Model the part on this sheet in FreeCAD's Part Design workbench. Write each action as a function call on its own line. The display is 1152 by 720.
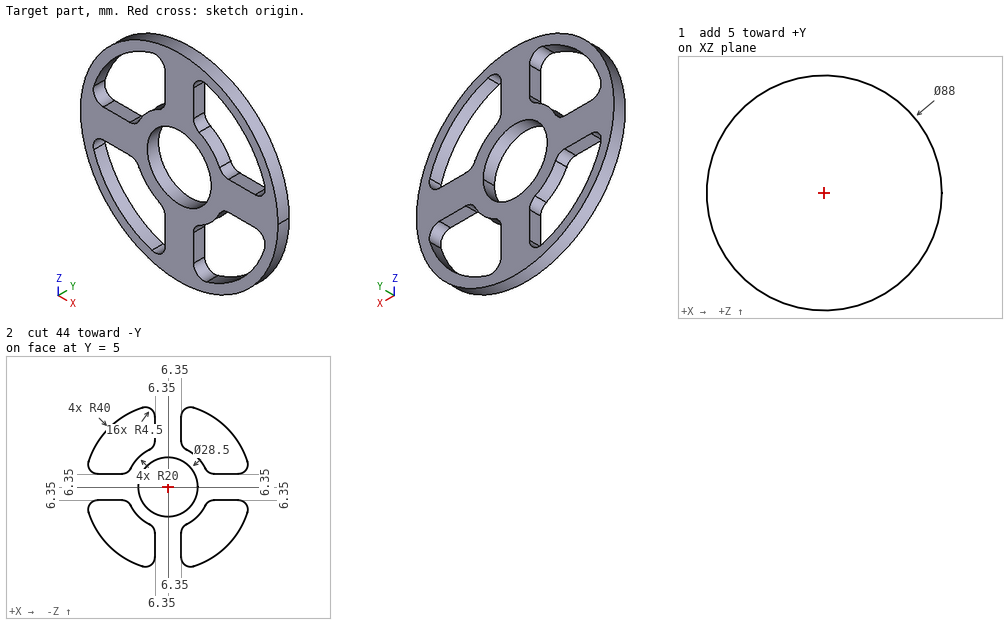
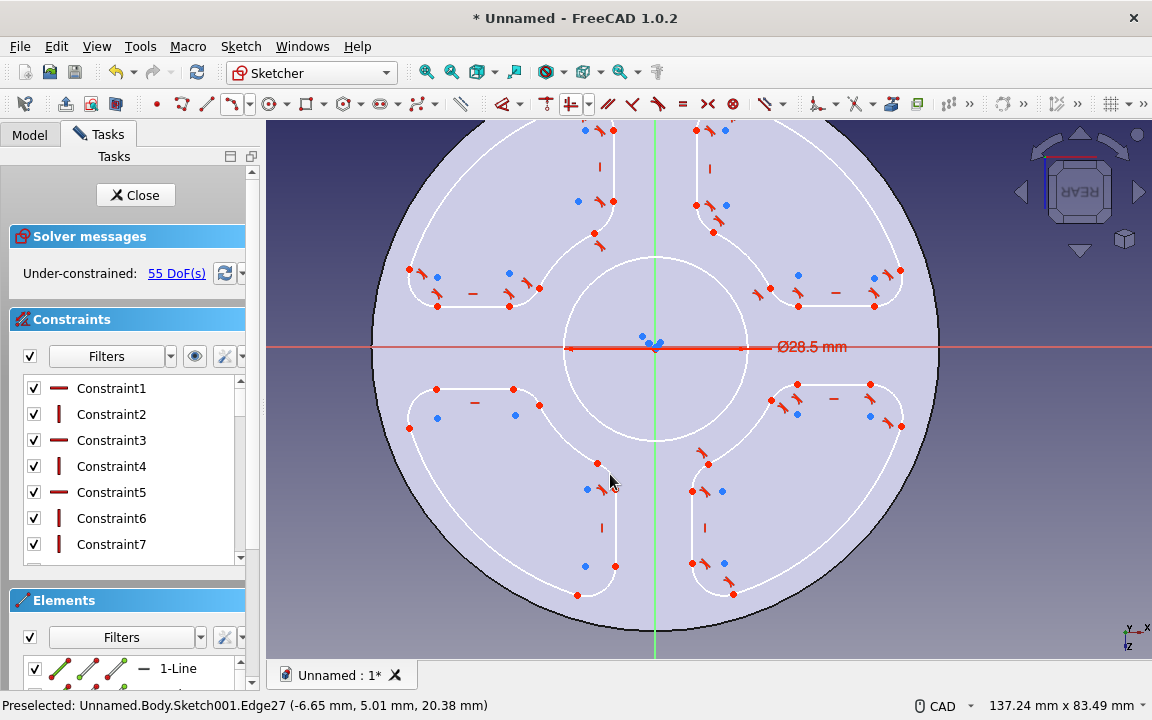
click(616, 543)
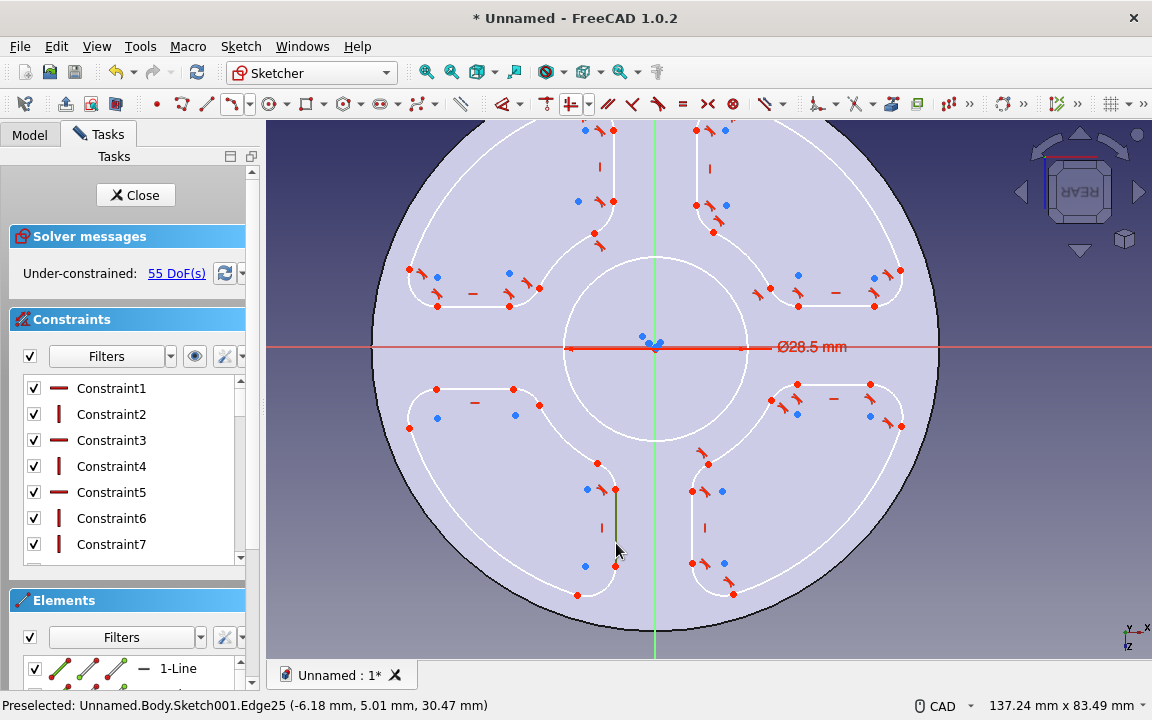
click(594, 595)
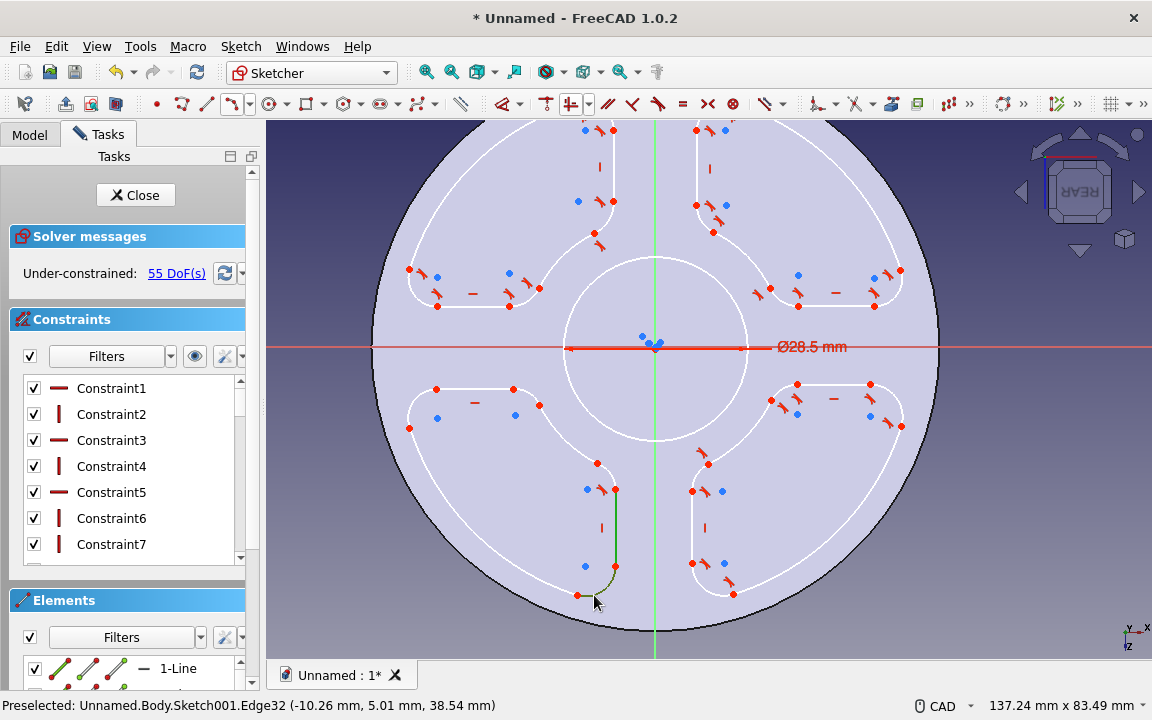
key(t)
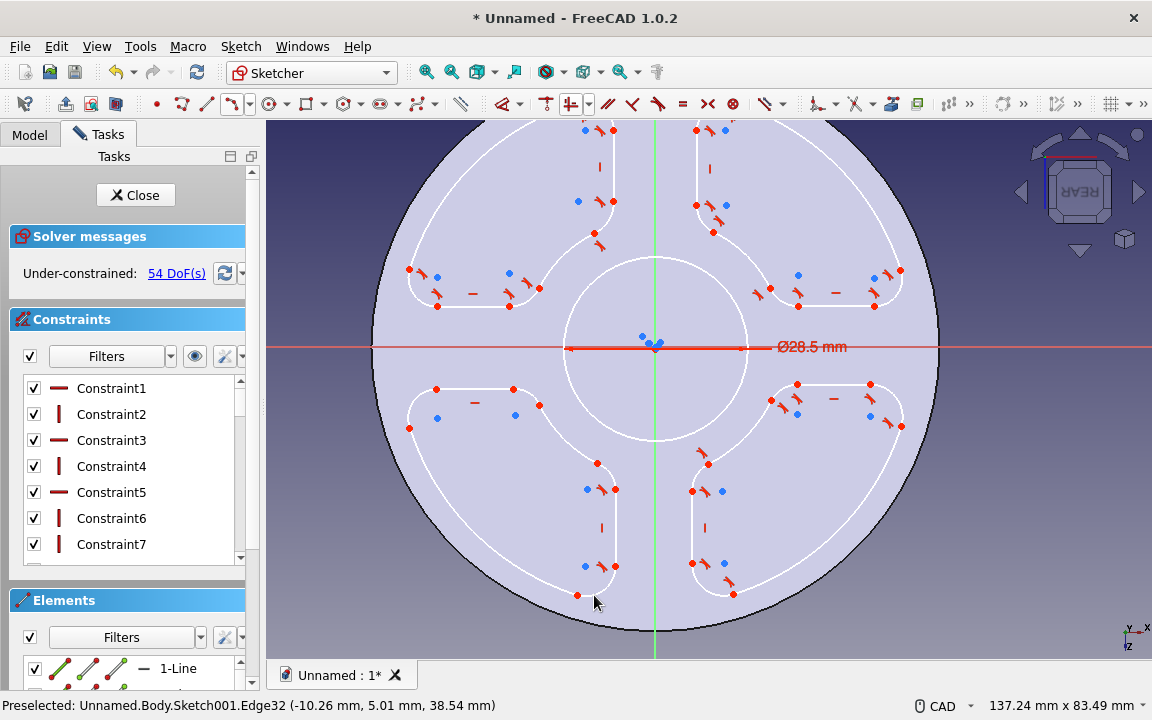
click(491, 389)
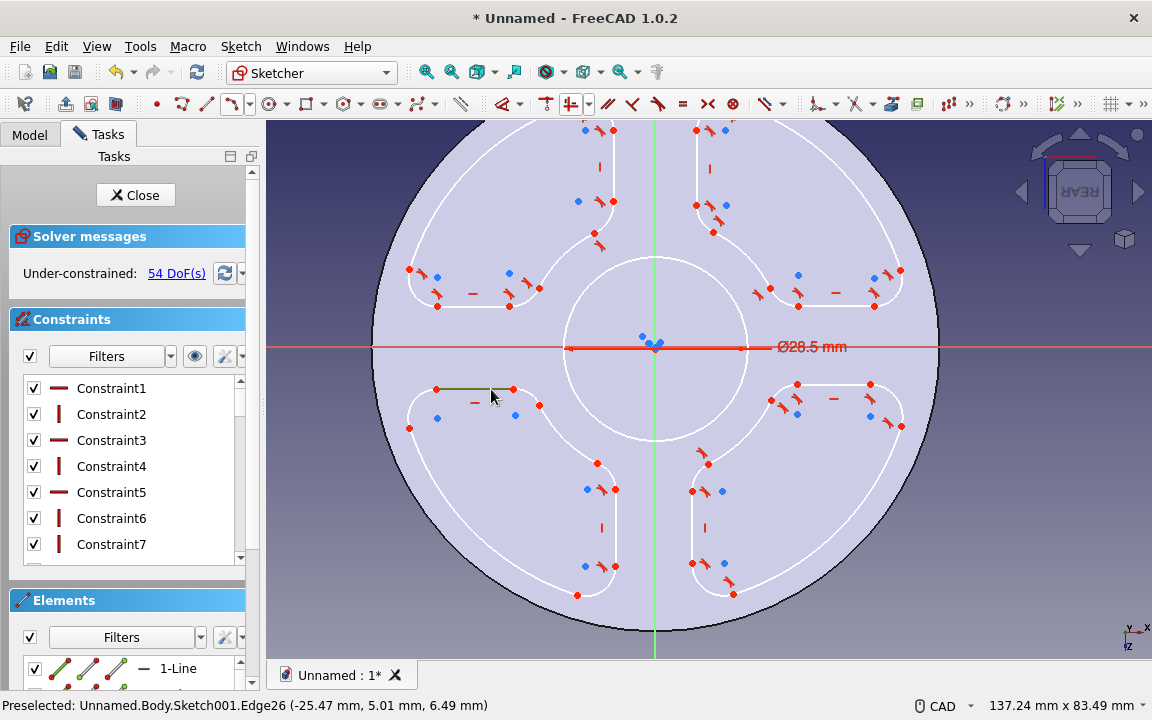
scroll(534, 397, up, 2)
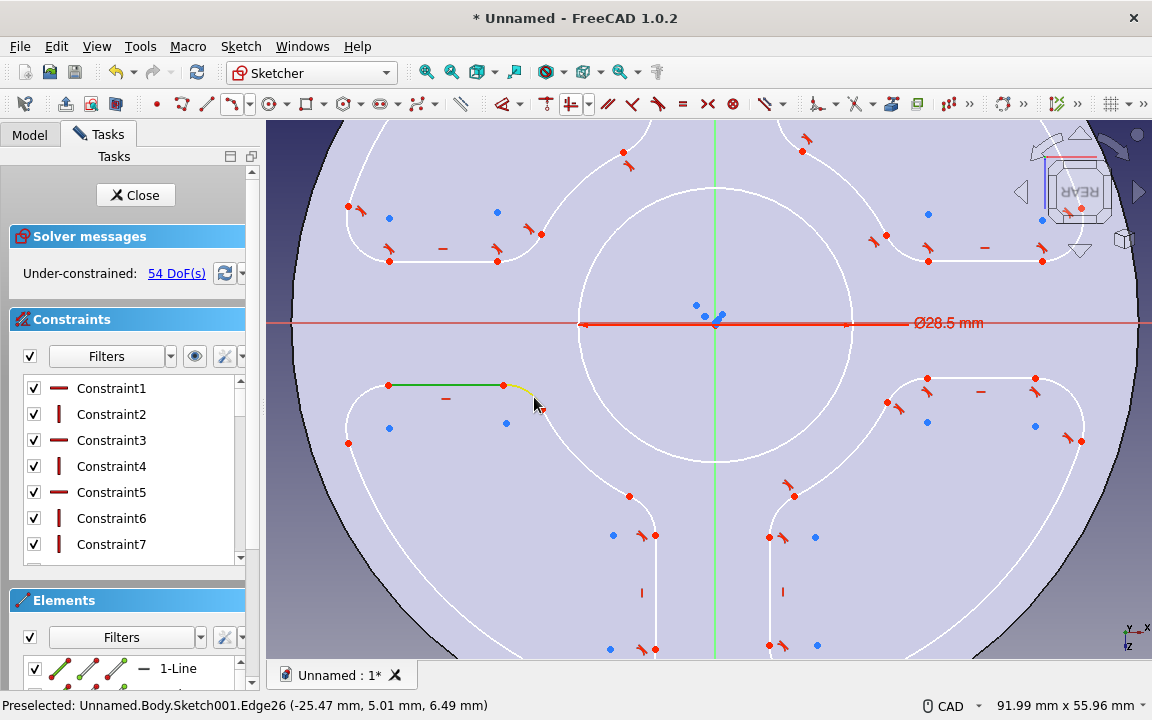
click(535, 397)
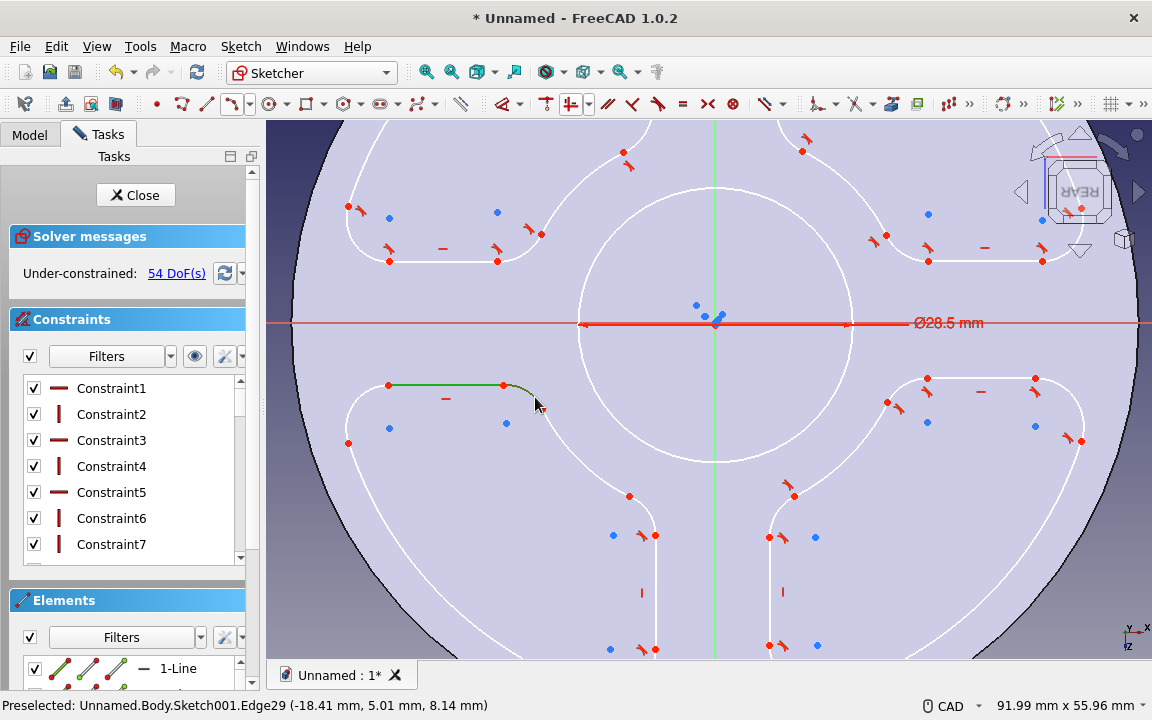
click(658, 104)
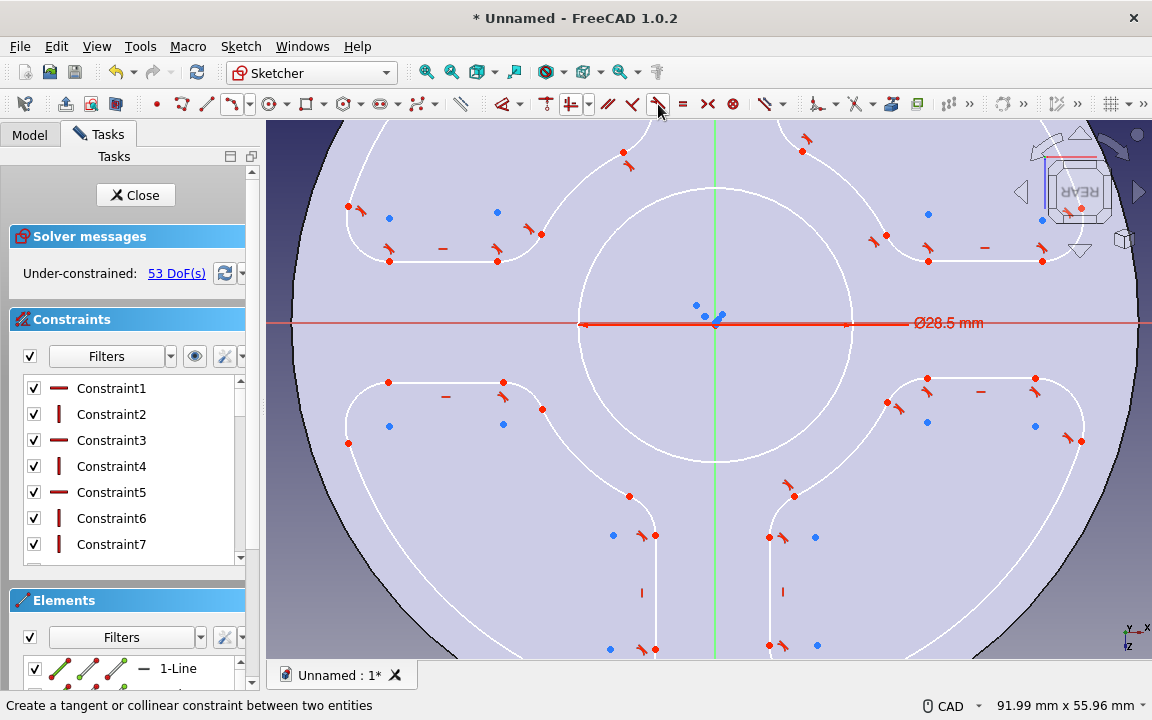
click(469, 383)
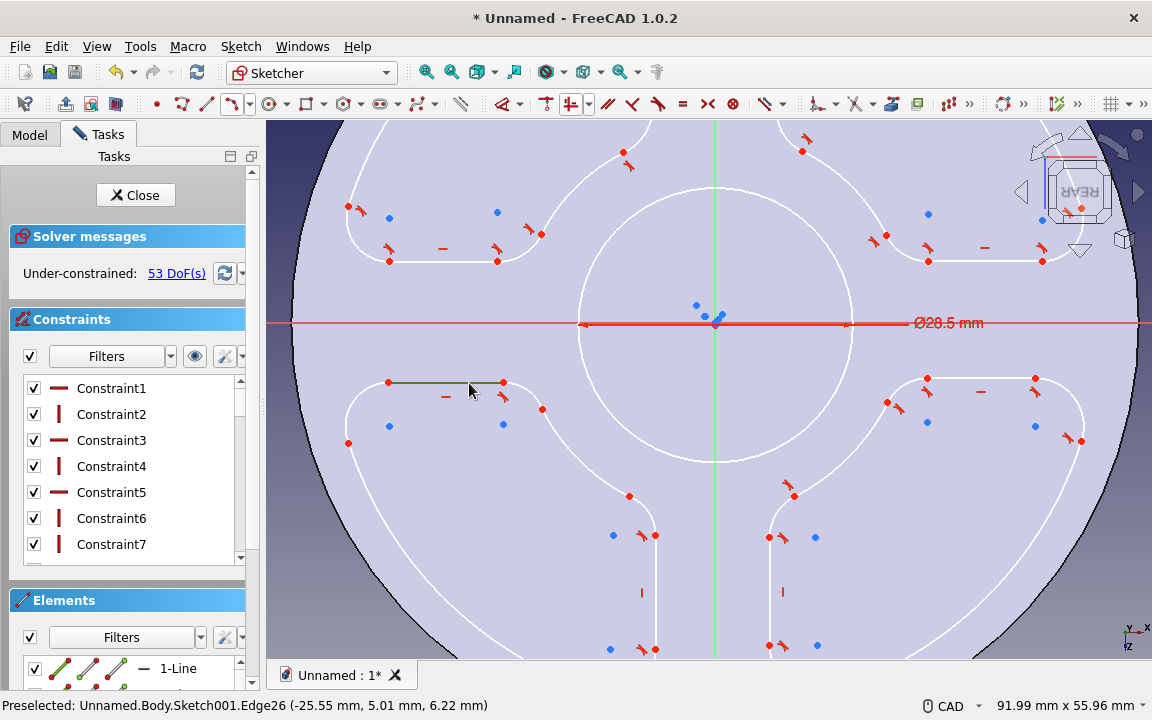
click(365, 390)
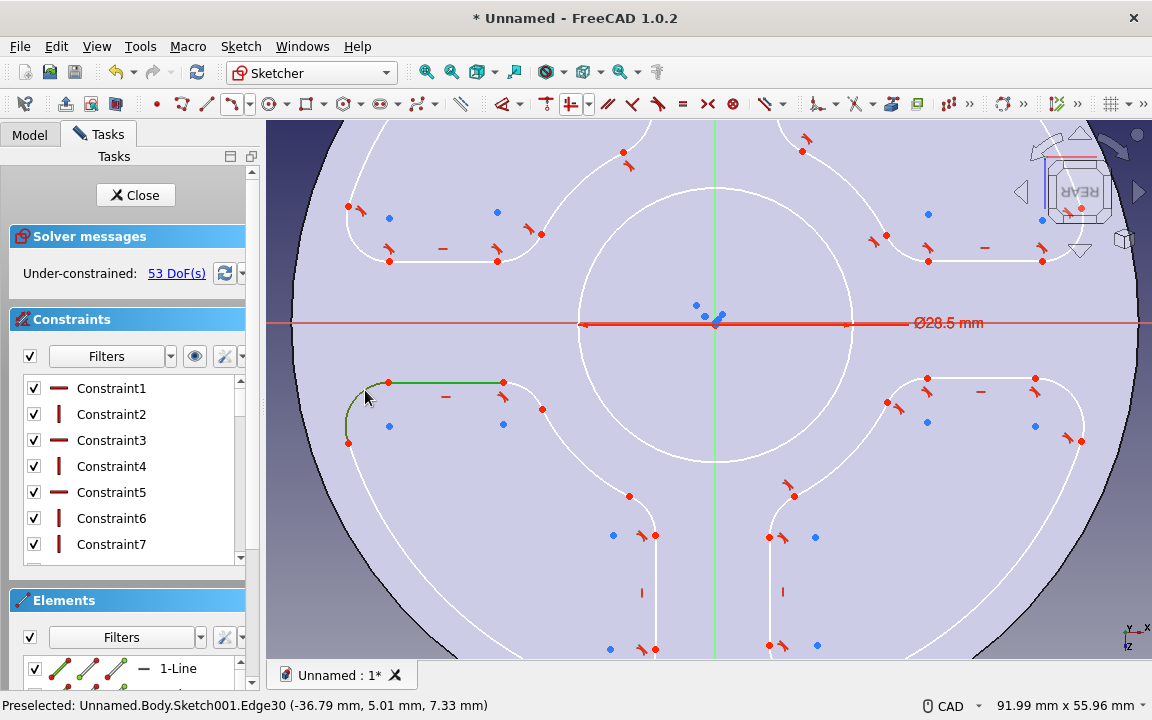
key(t)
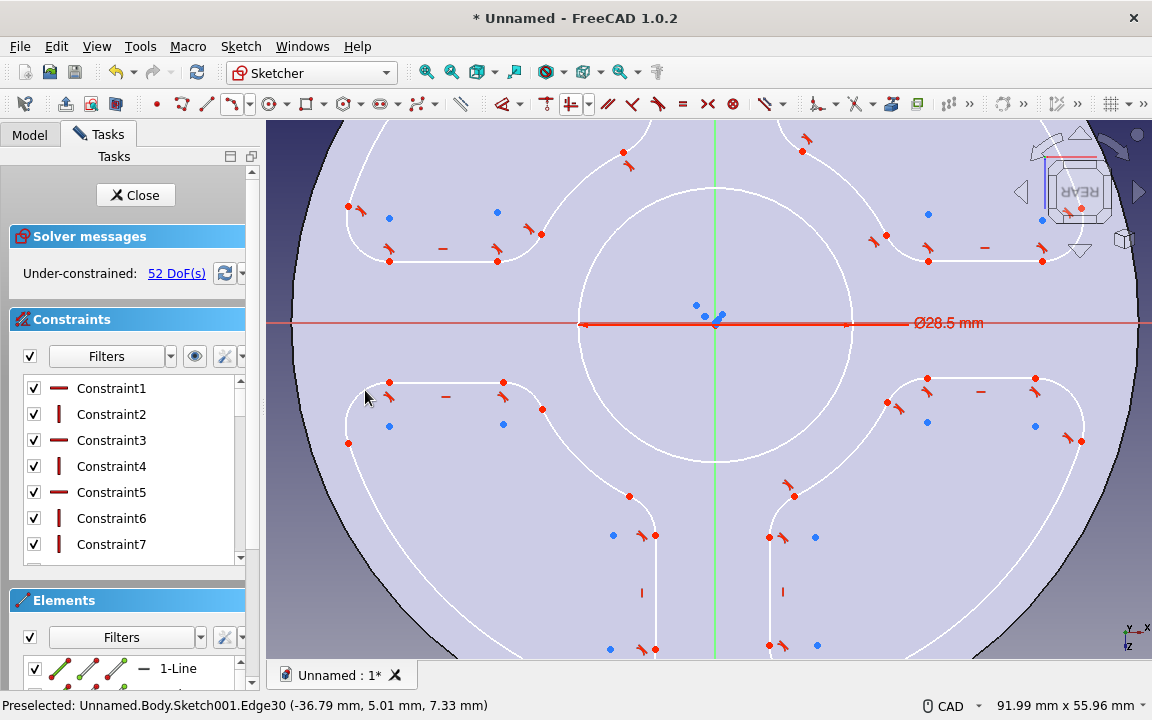
click(653, 521)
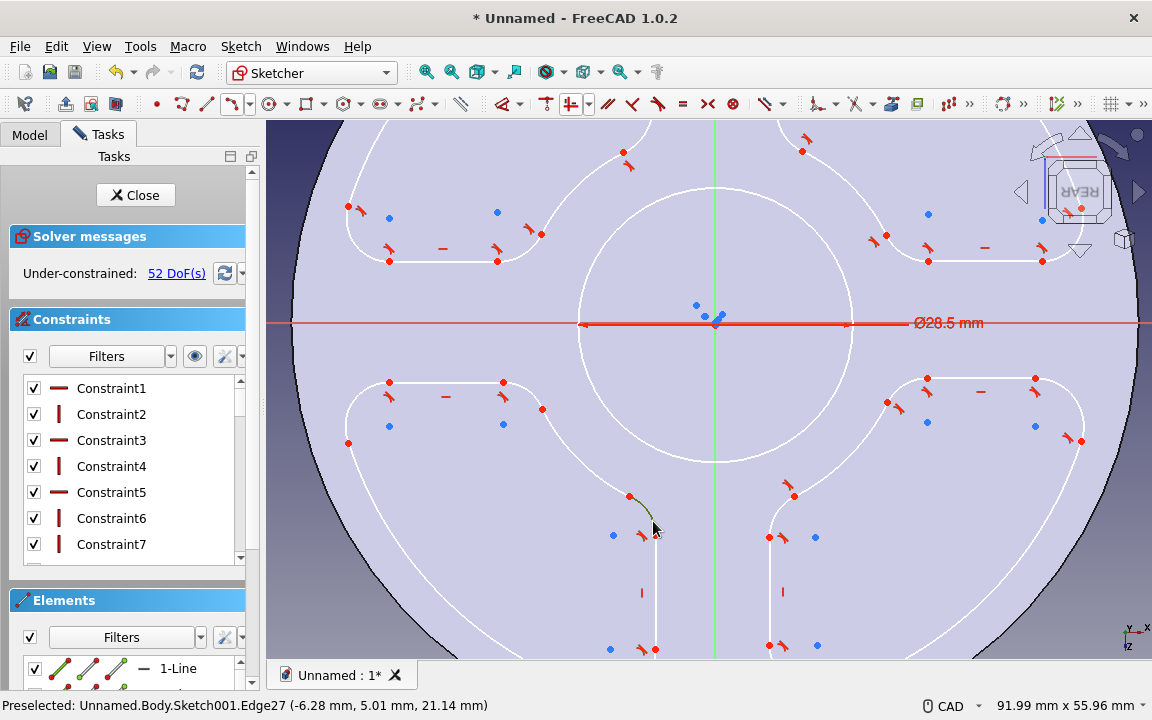
click(562, 441)